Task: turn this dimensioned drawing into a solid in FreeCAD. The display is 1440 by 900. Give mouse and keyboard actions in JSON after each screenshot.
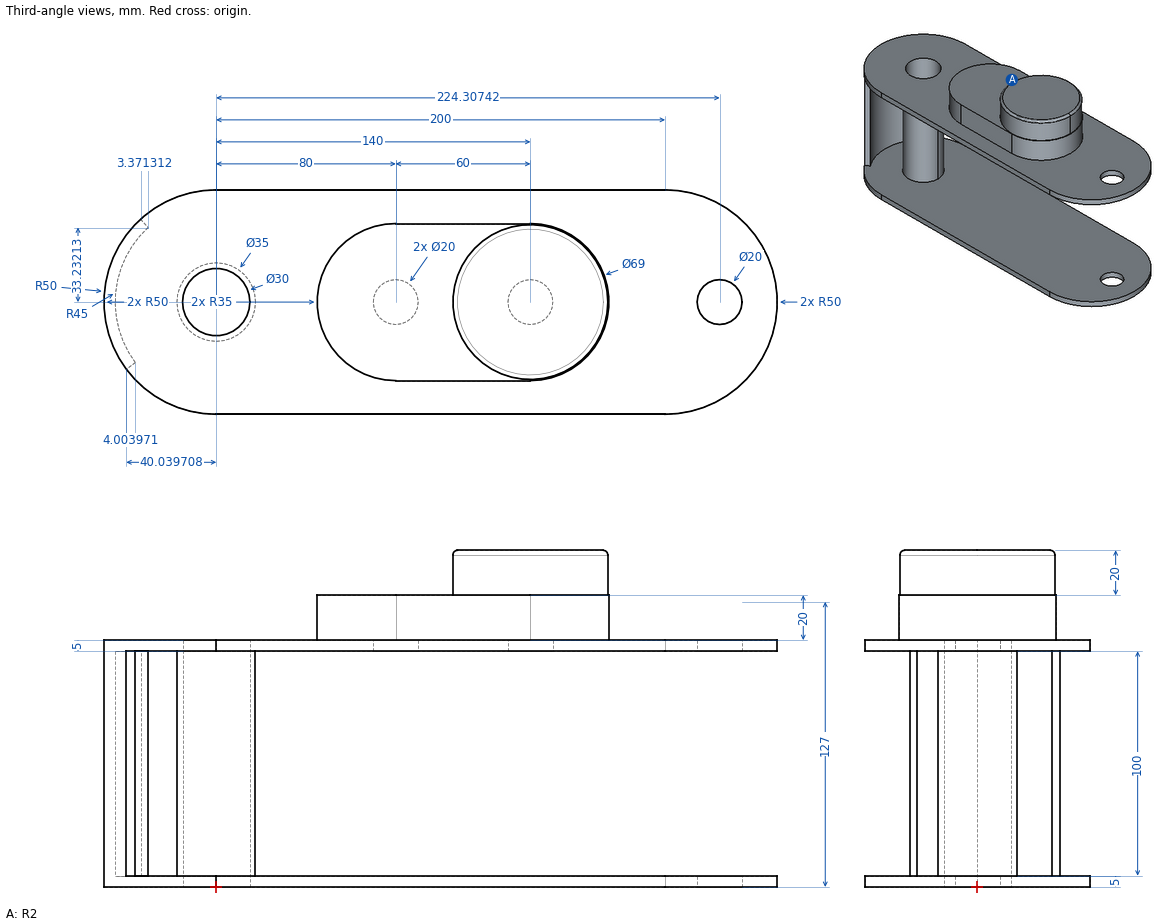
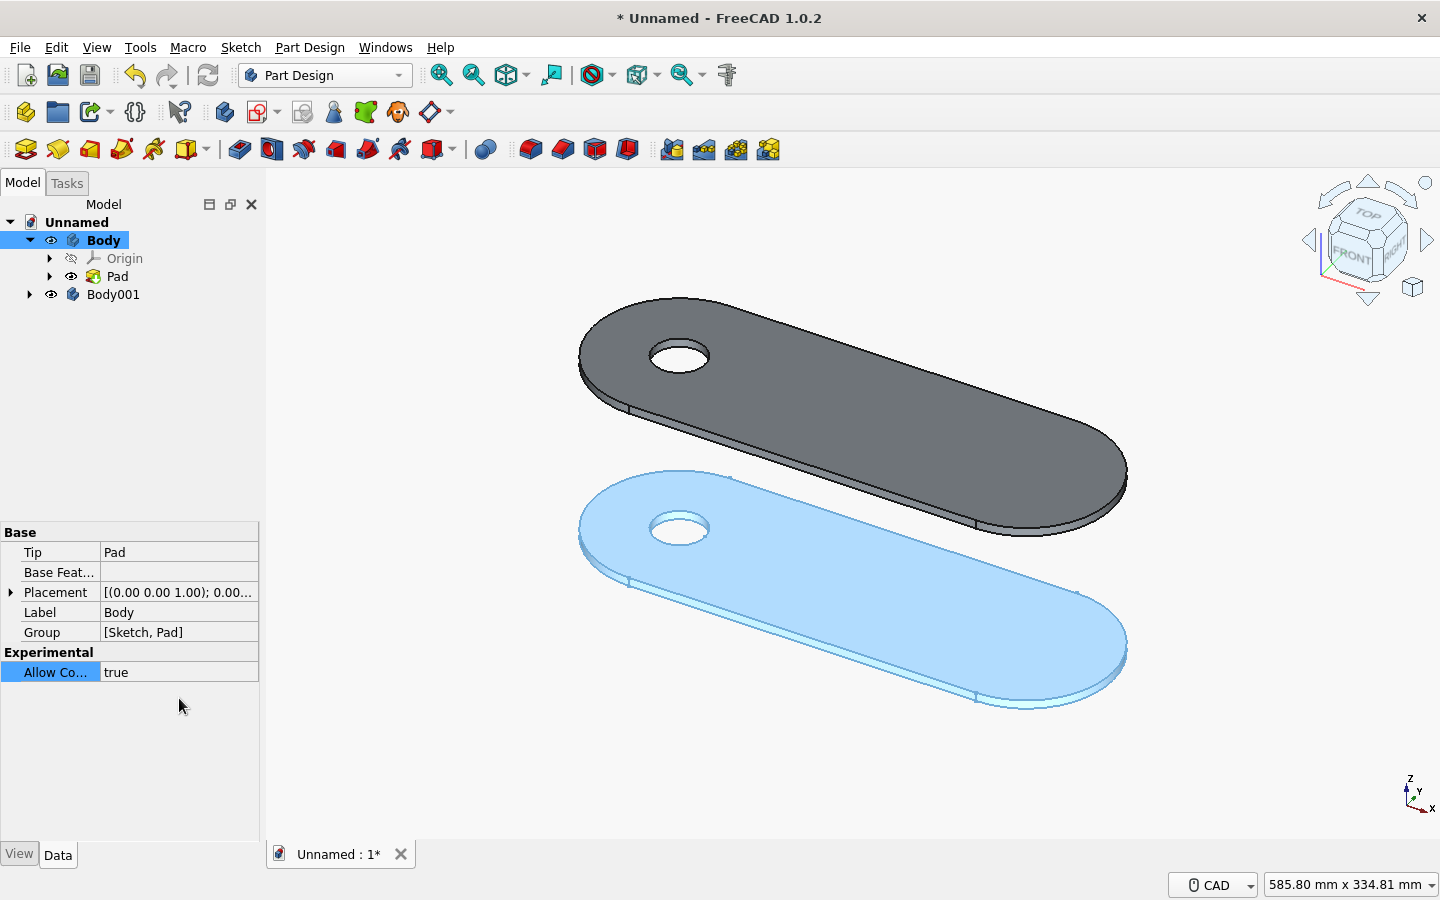
{"action": "left_click", "coordinate": [96, 294]}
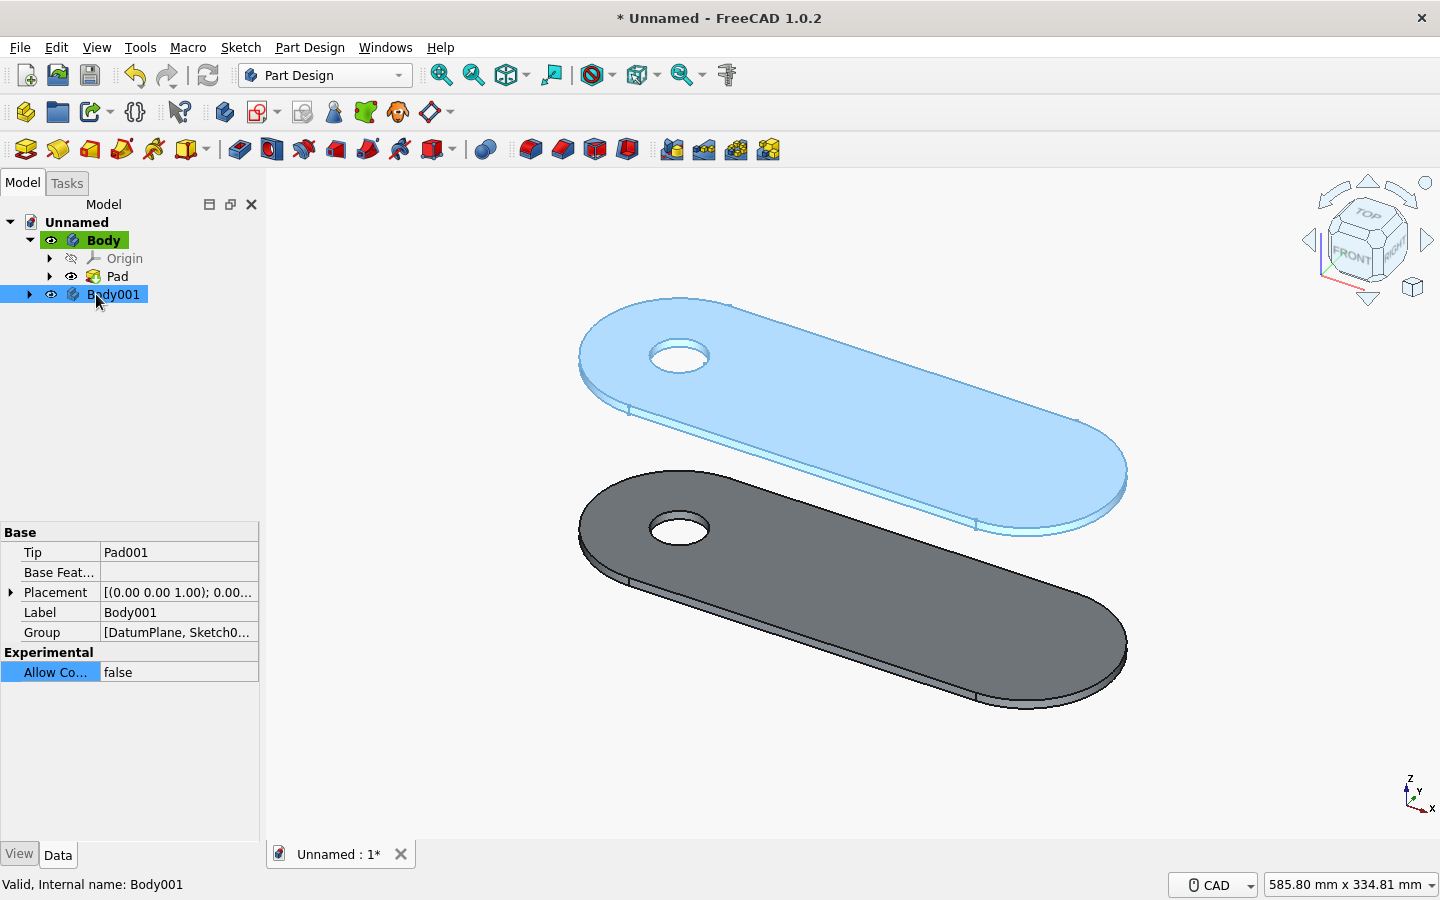
{"action": "left_click", "coordinate": [486, 150]}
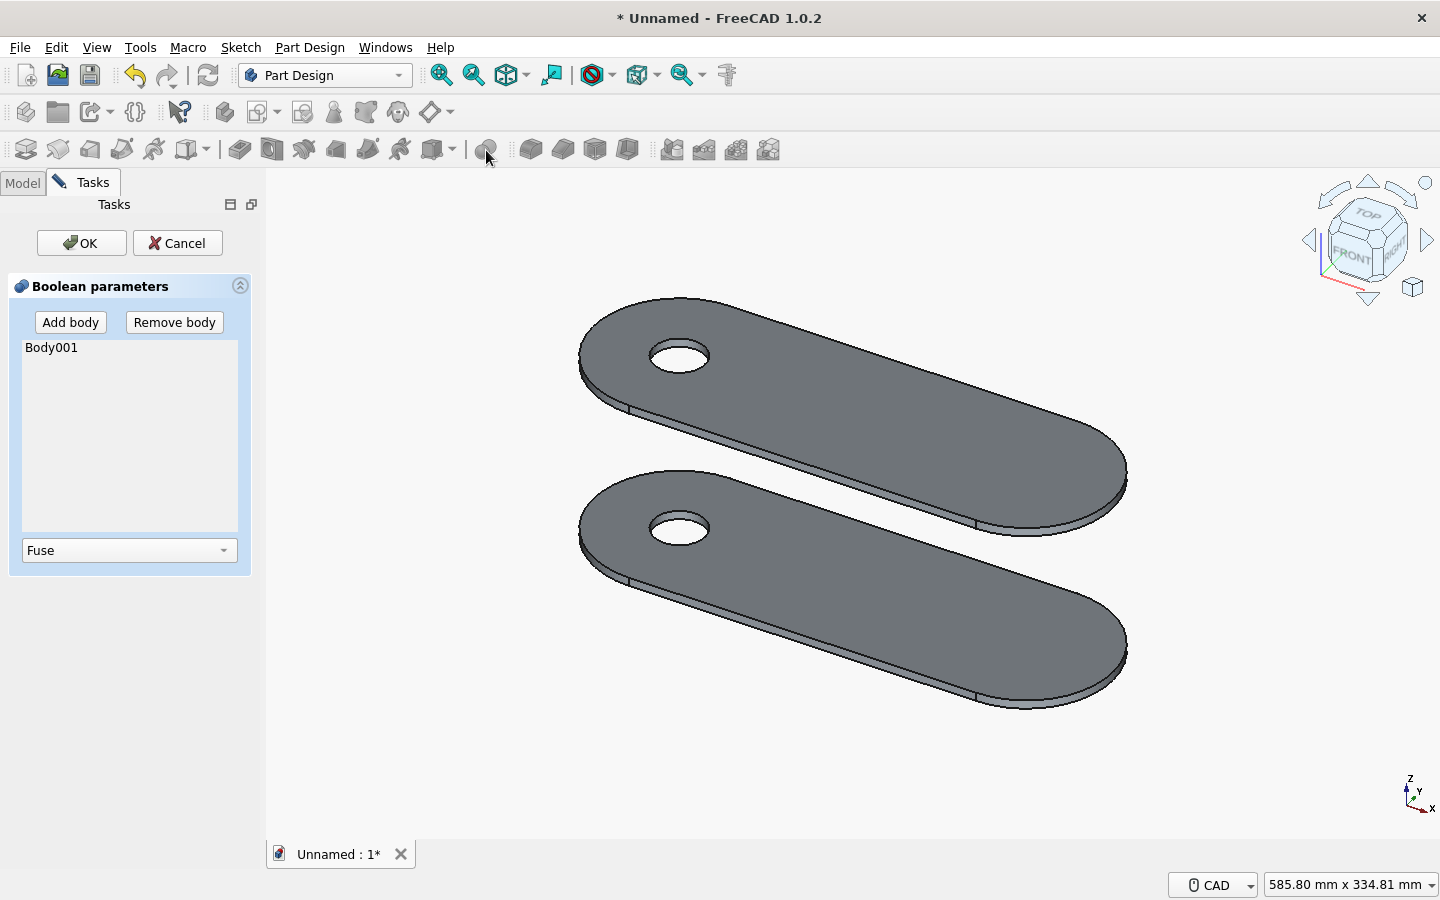
{"action": "left_click", "coordinate": [82, 243]}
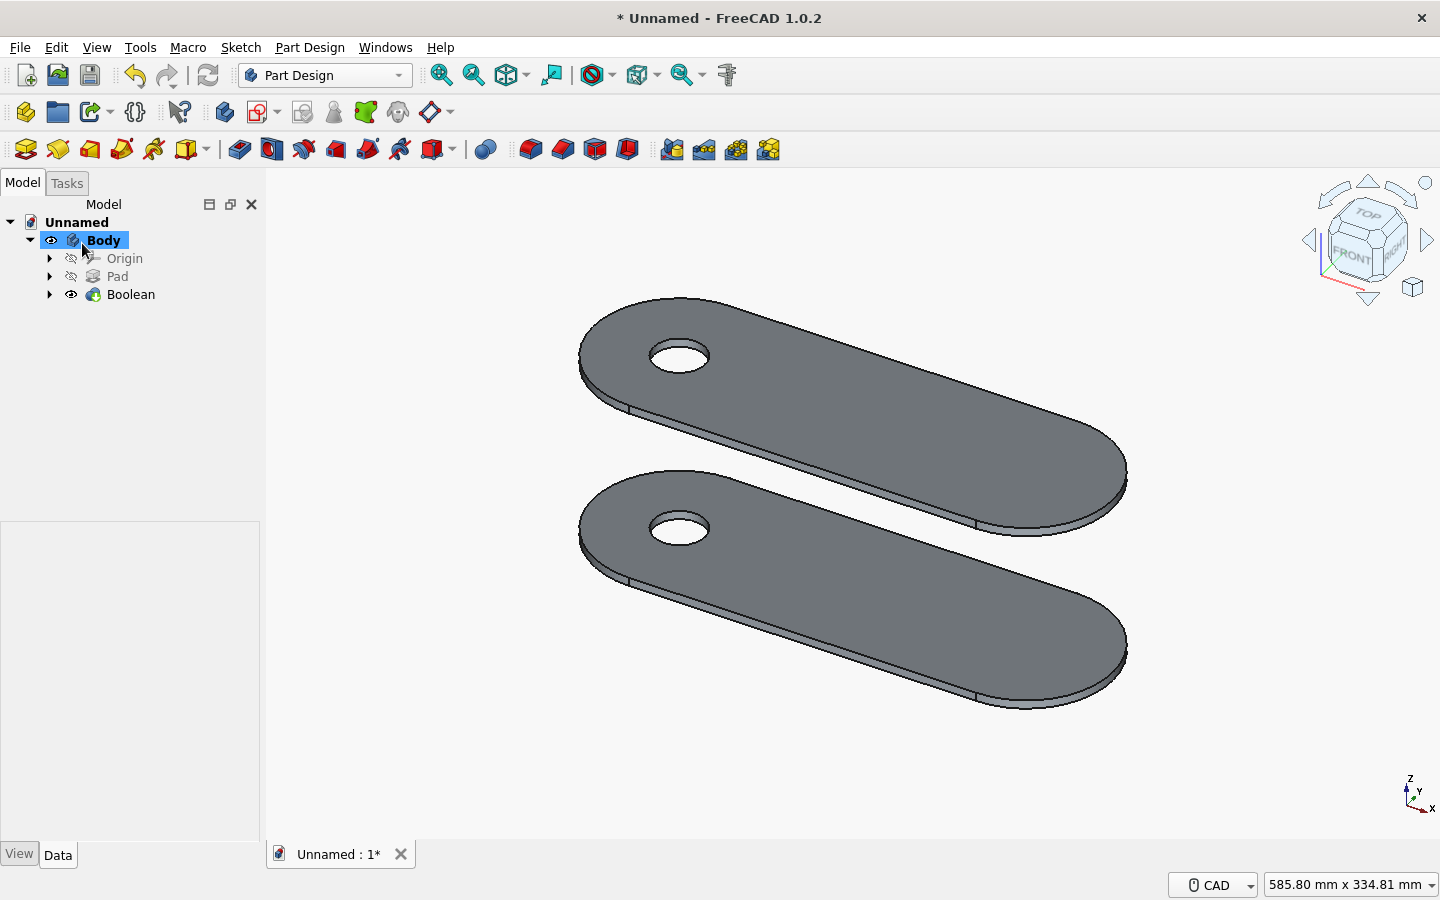
{"action": "left_click", "coordinate": [50, 258]}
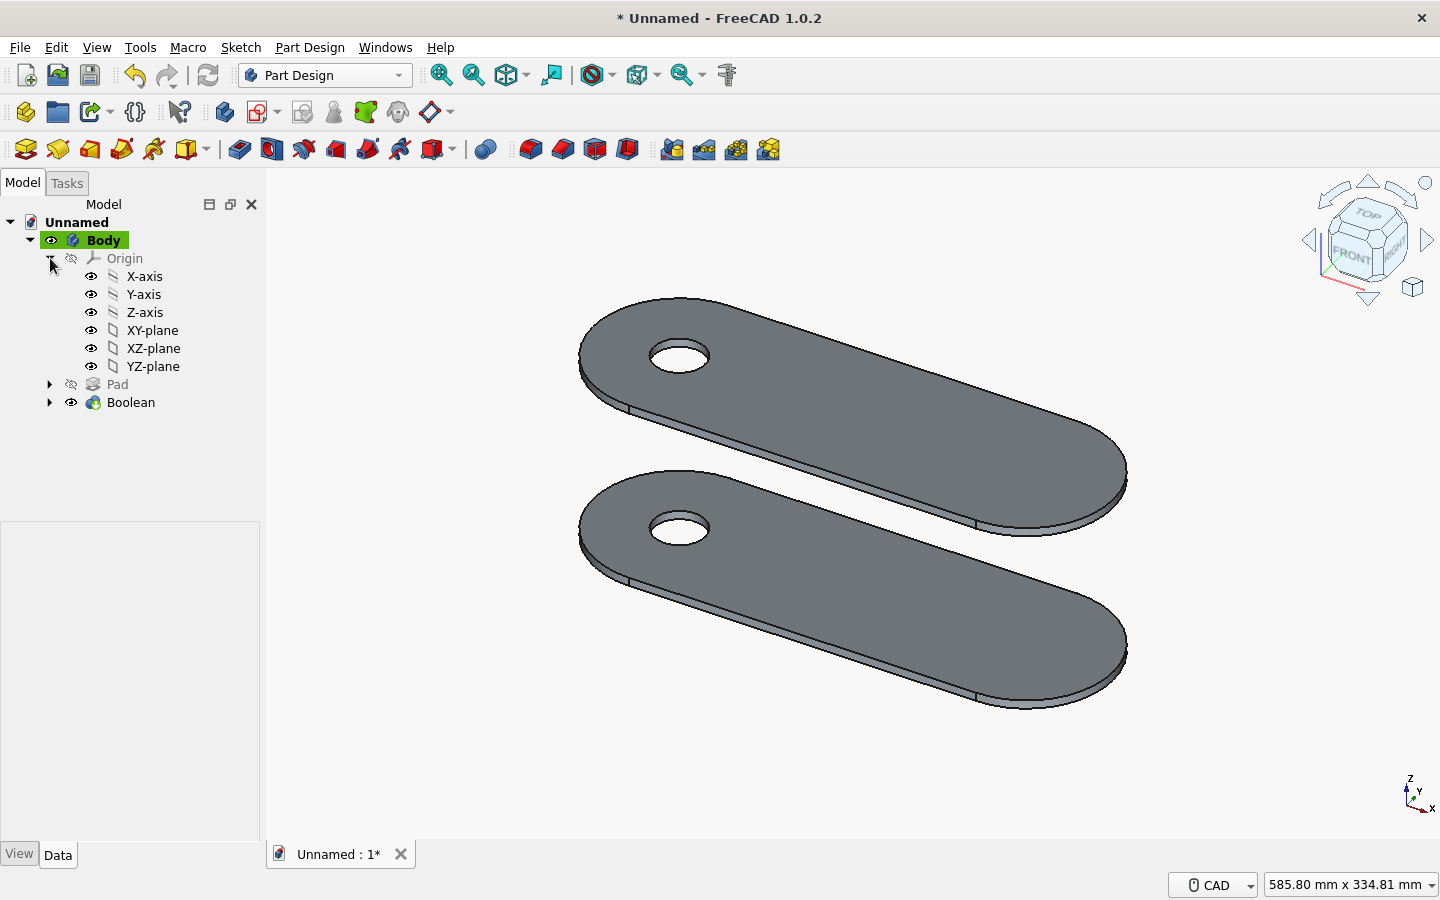
{"action": "left_click", "coordinate": [136, 330]}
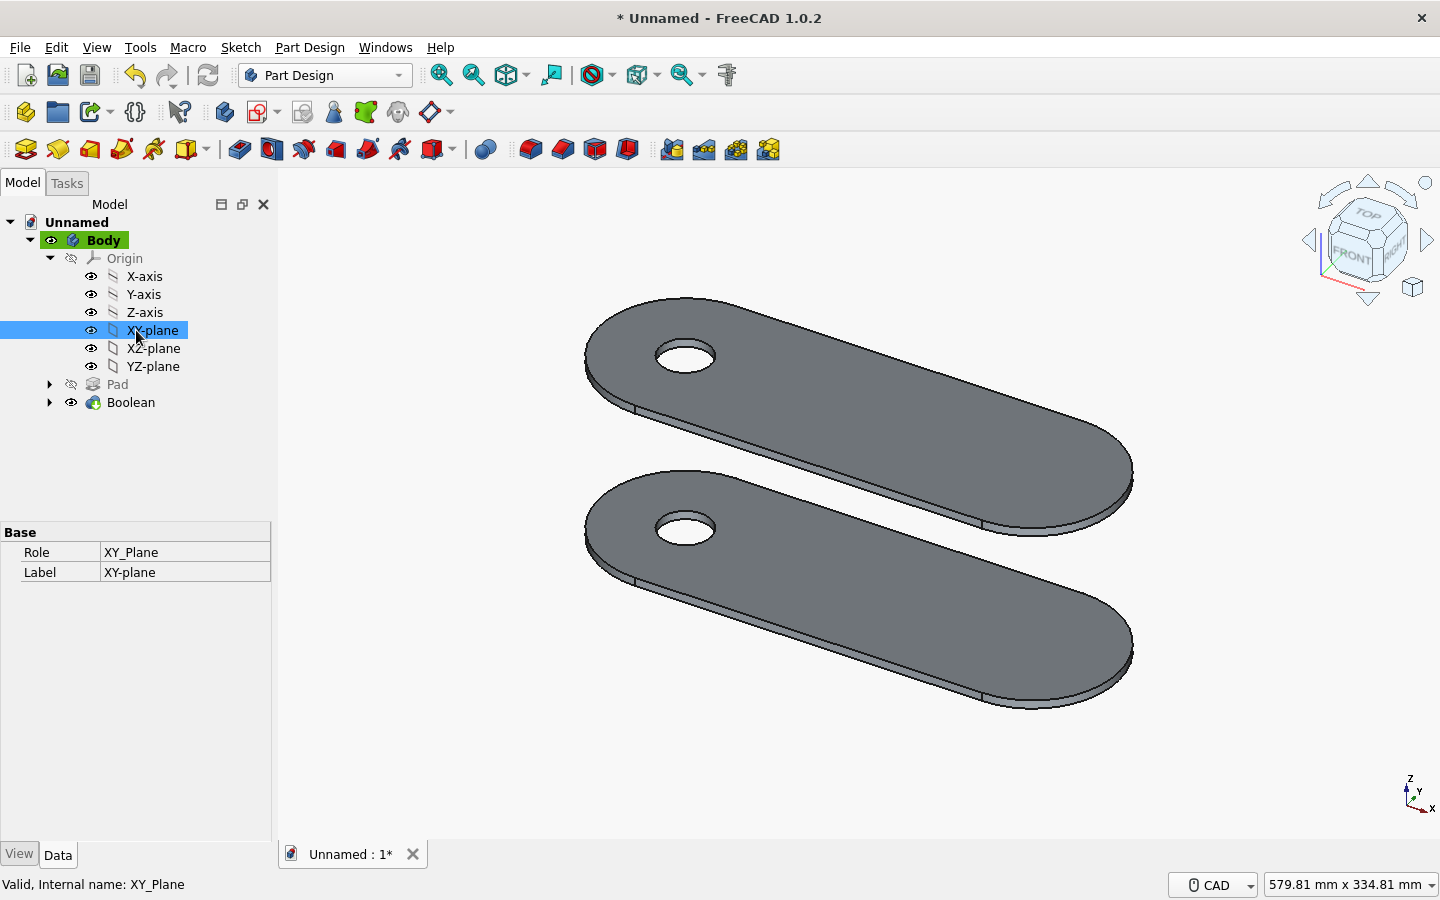
{"action": "left_click", "coordinate": [430, 112]}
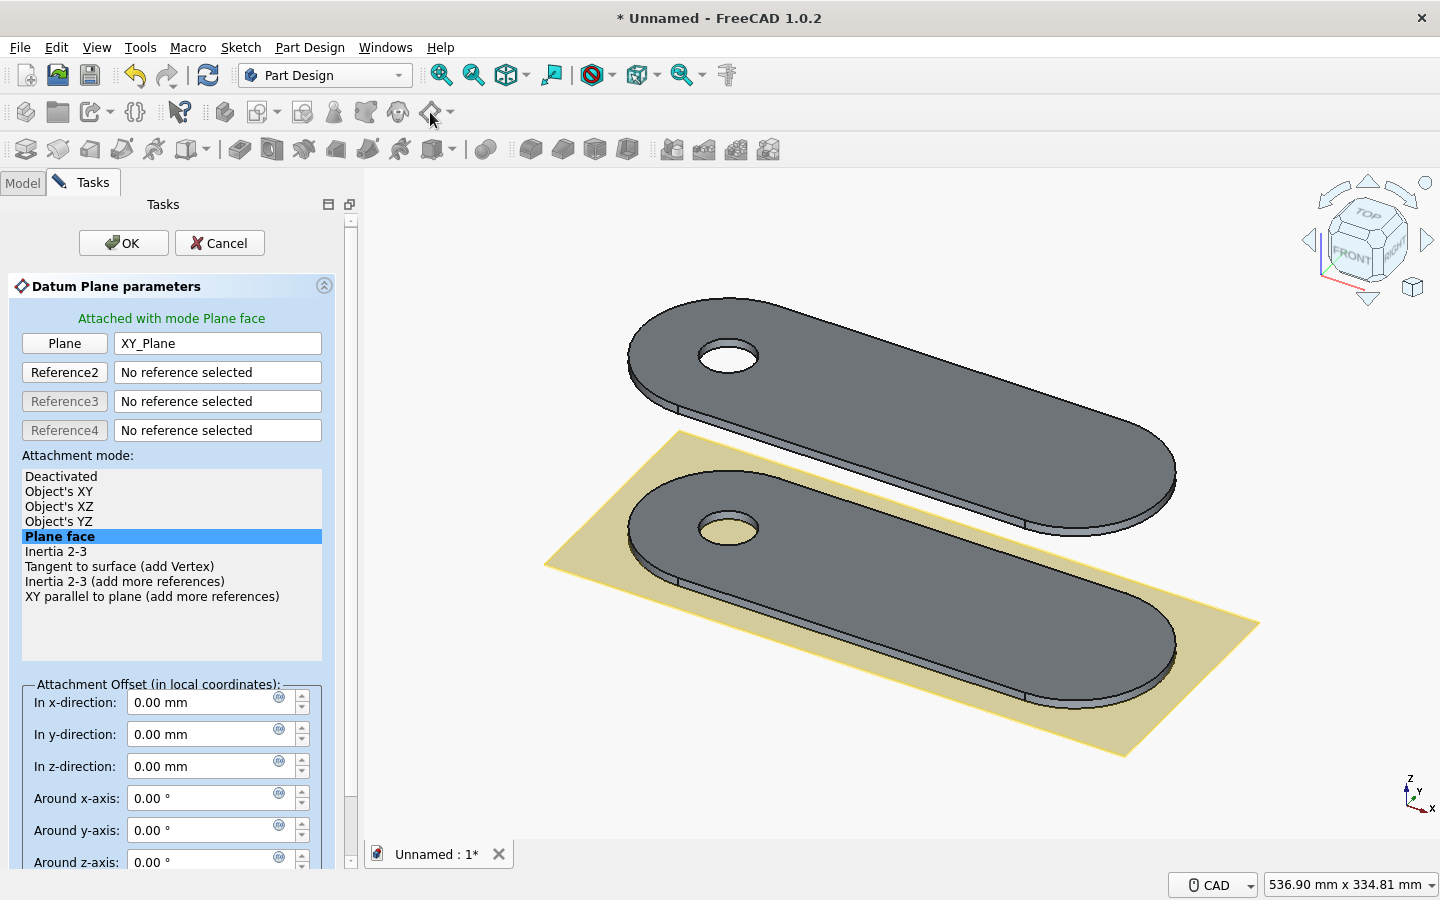
{"action": "triple_click", "coordinate": [210, 766]}